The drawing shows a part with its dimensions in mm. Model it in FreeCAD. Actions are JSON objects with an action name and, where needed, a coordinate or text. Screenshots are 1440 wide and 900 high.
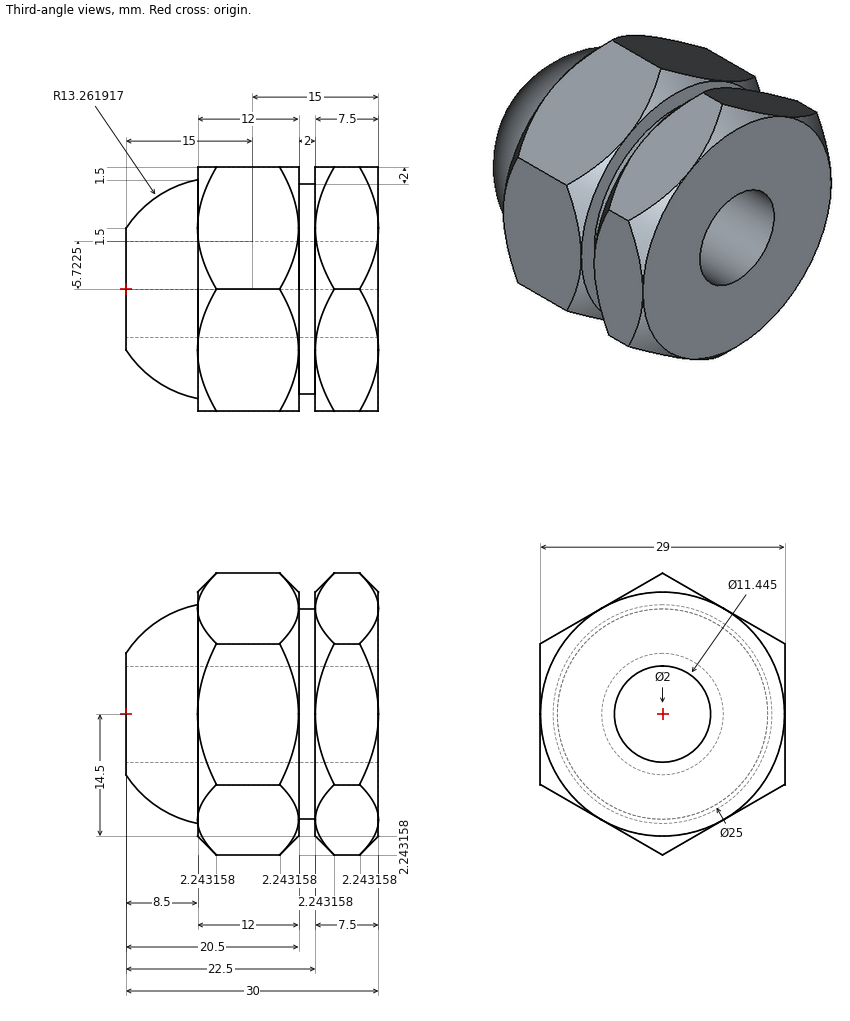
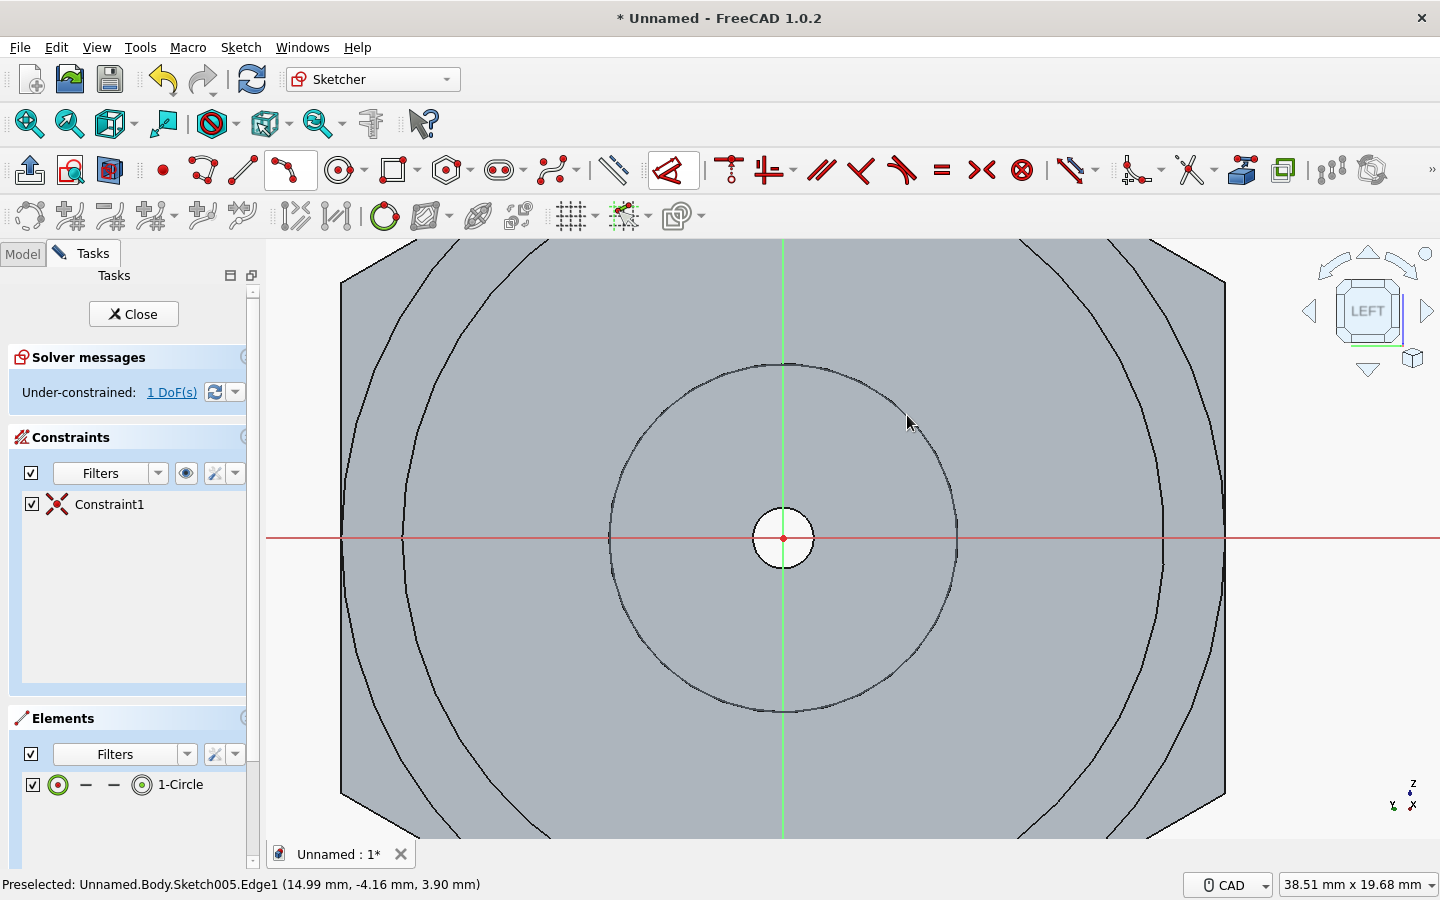
{"action": "left_click", "coordinate": [906, 415]}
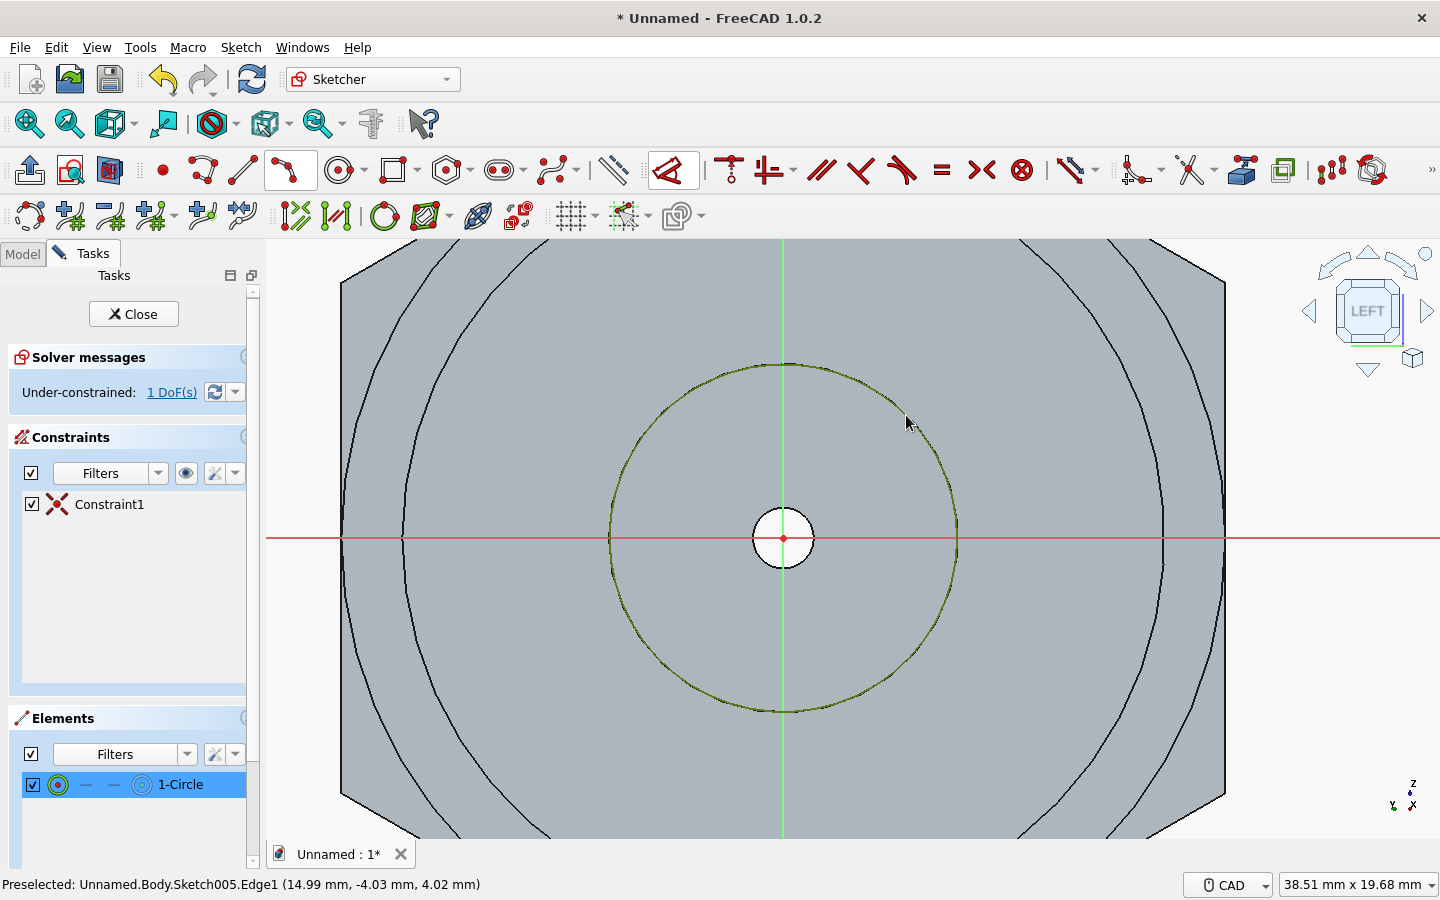
{"action": "left_click", "coordinate": [694, 170]}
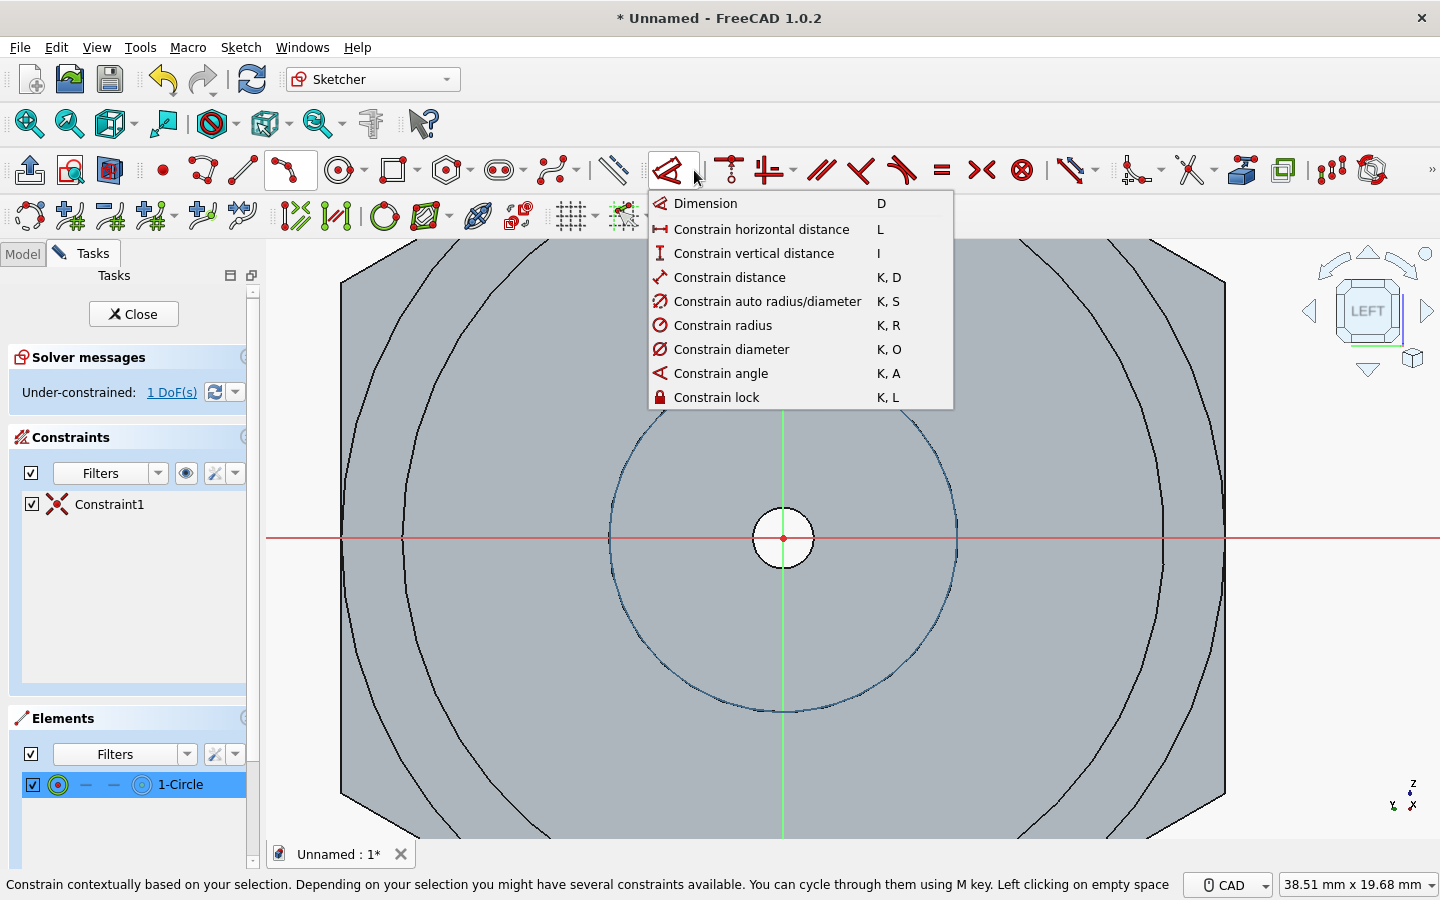
{"action": "left_click", "coordinate": [801, 349]}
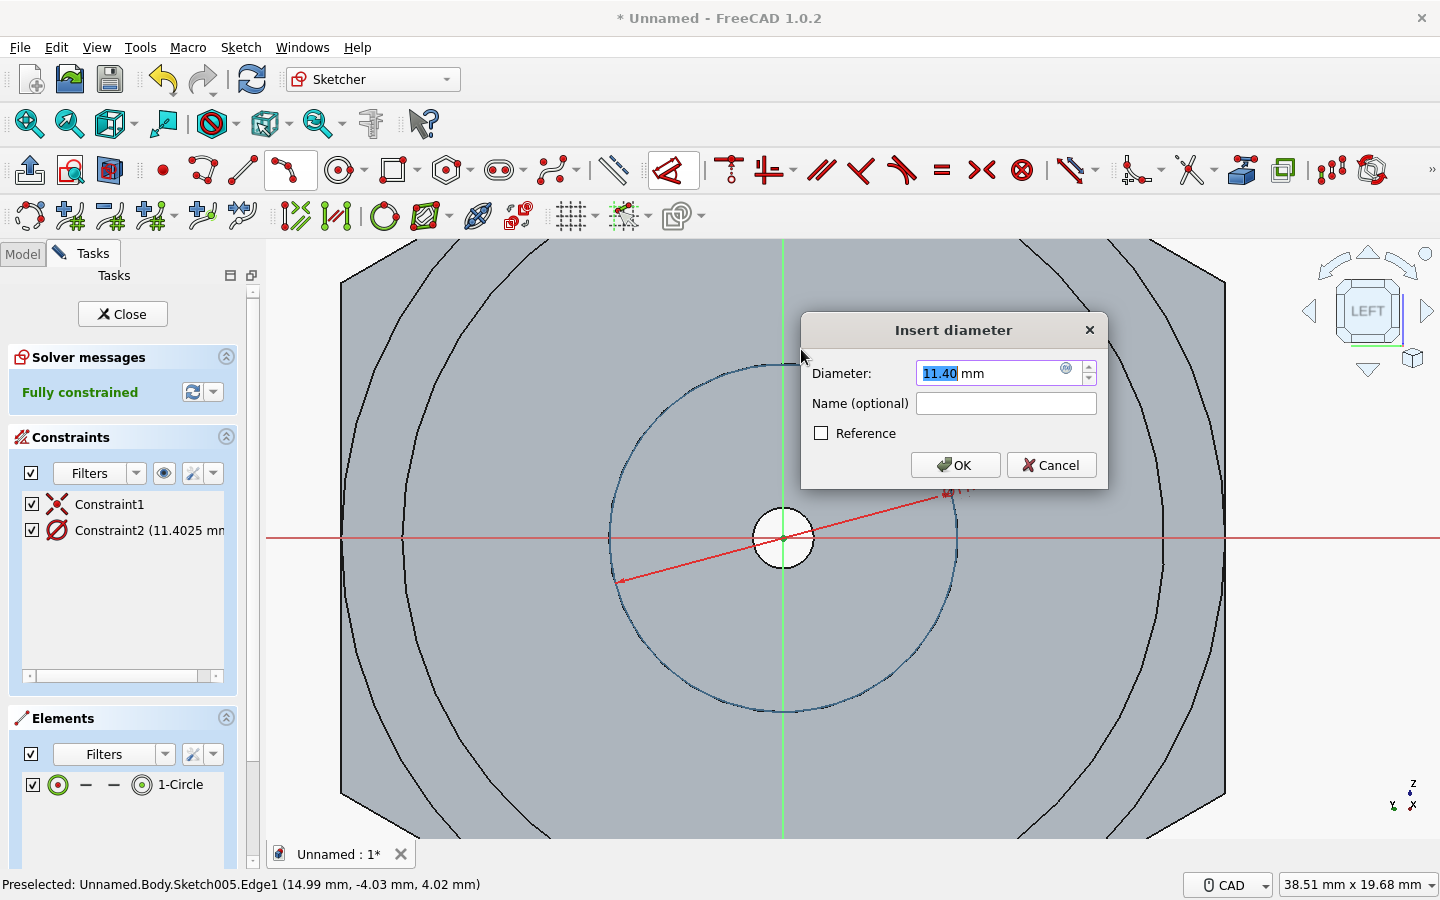
{"action": "type", "text": "11.445"}
{"action": "key", "text": "Return"}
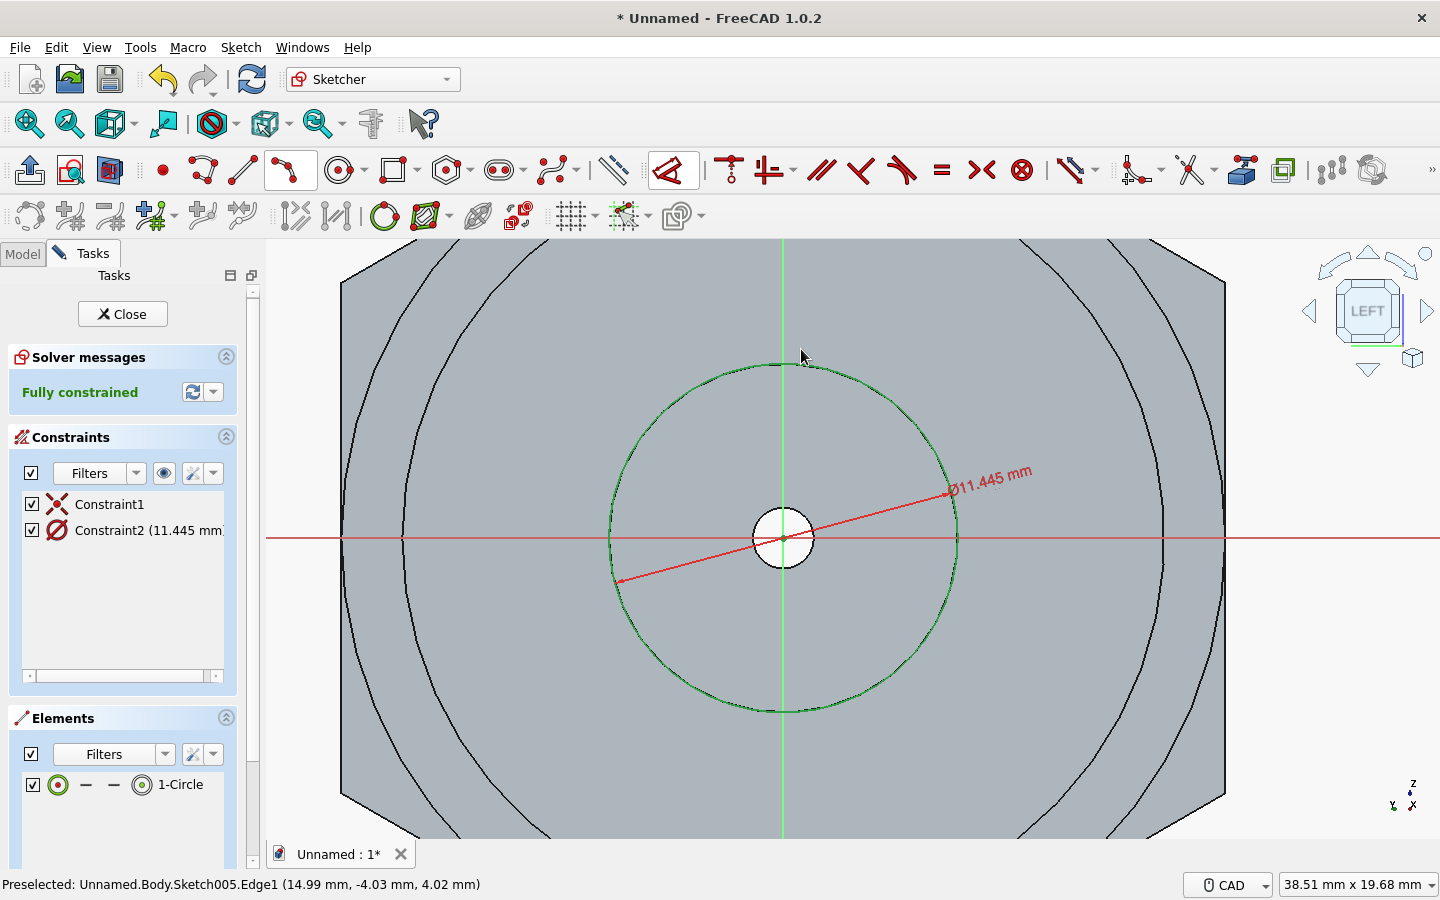
{"action": "left_click", "coordinate": [123, 314]}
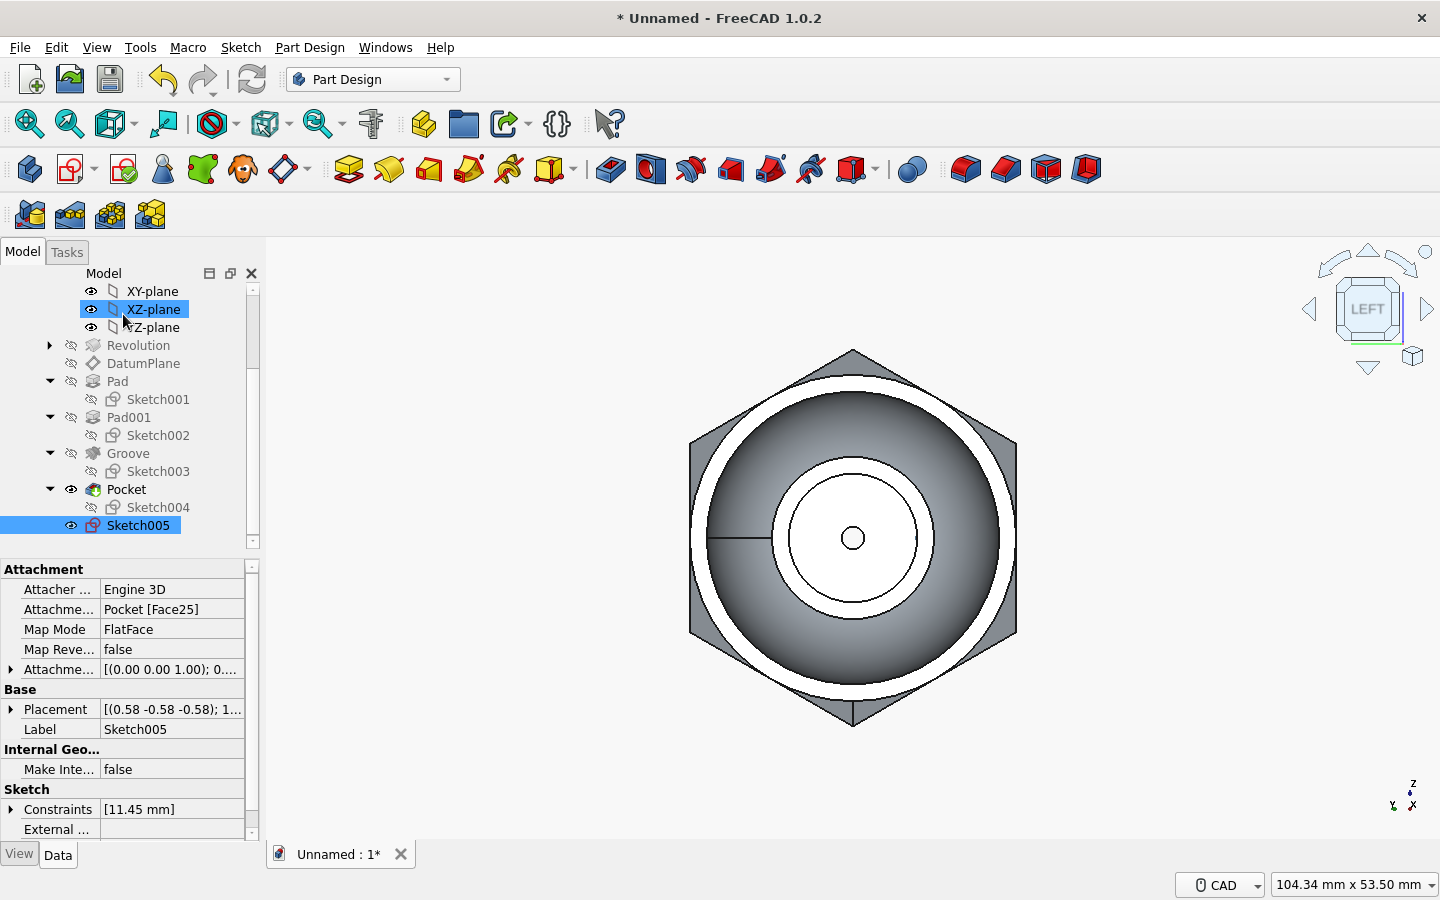
{"action": "left_click", "coordinate": [612, 170]}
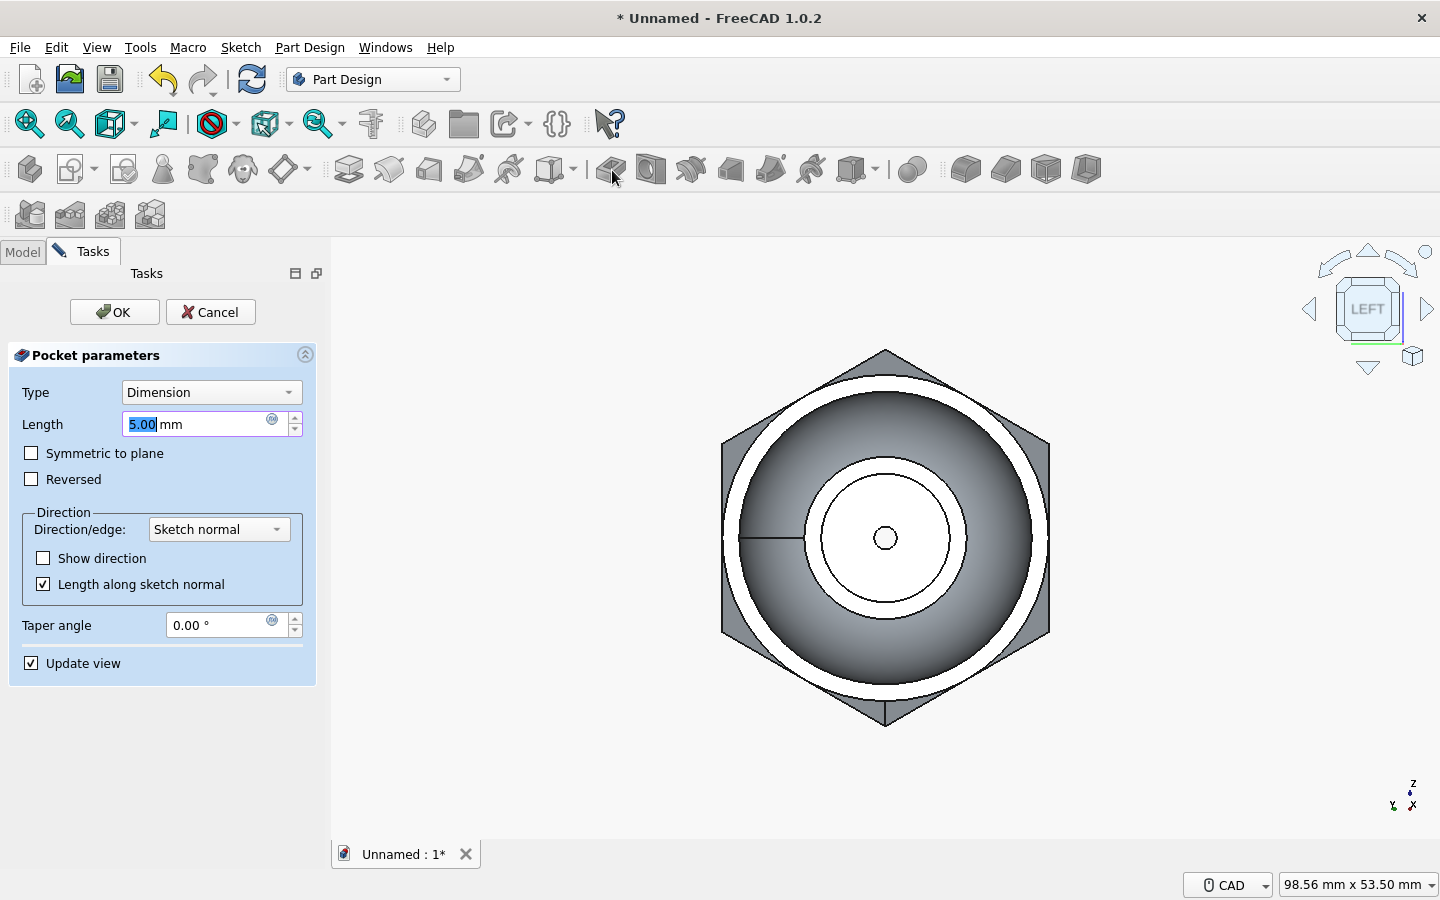
{"action": "type", "text": "15"}
{"action": "key", "text": "Tab"}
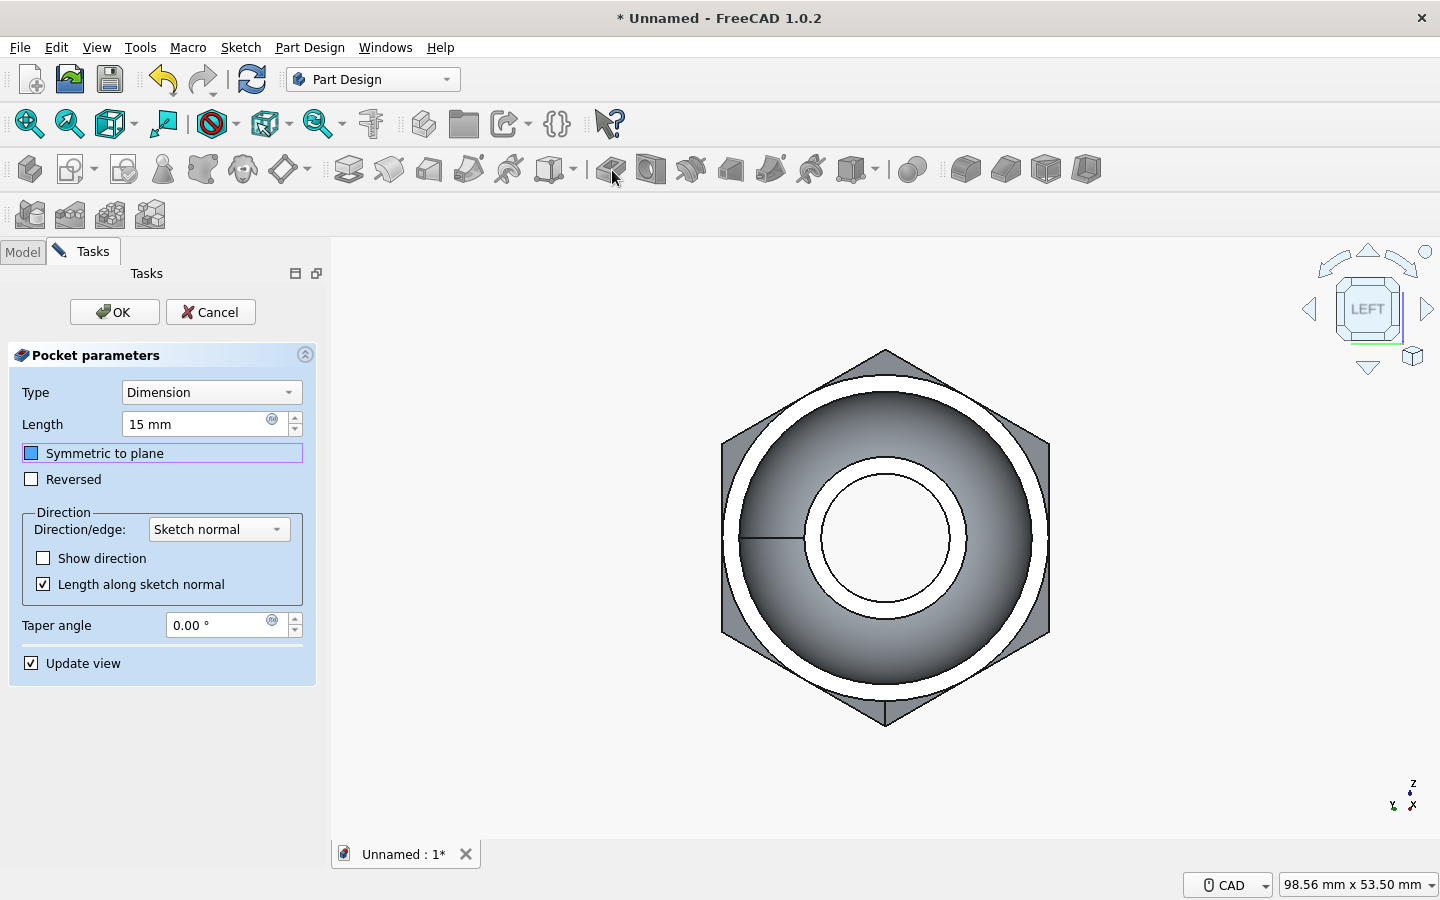
{"action": "left_click", "coordinate": [115, 312]}